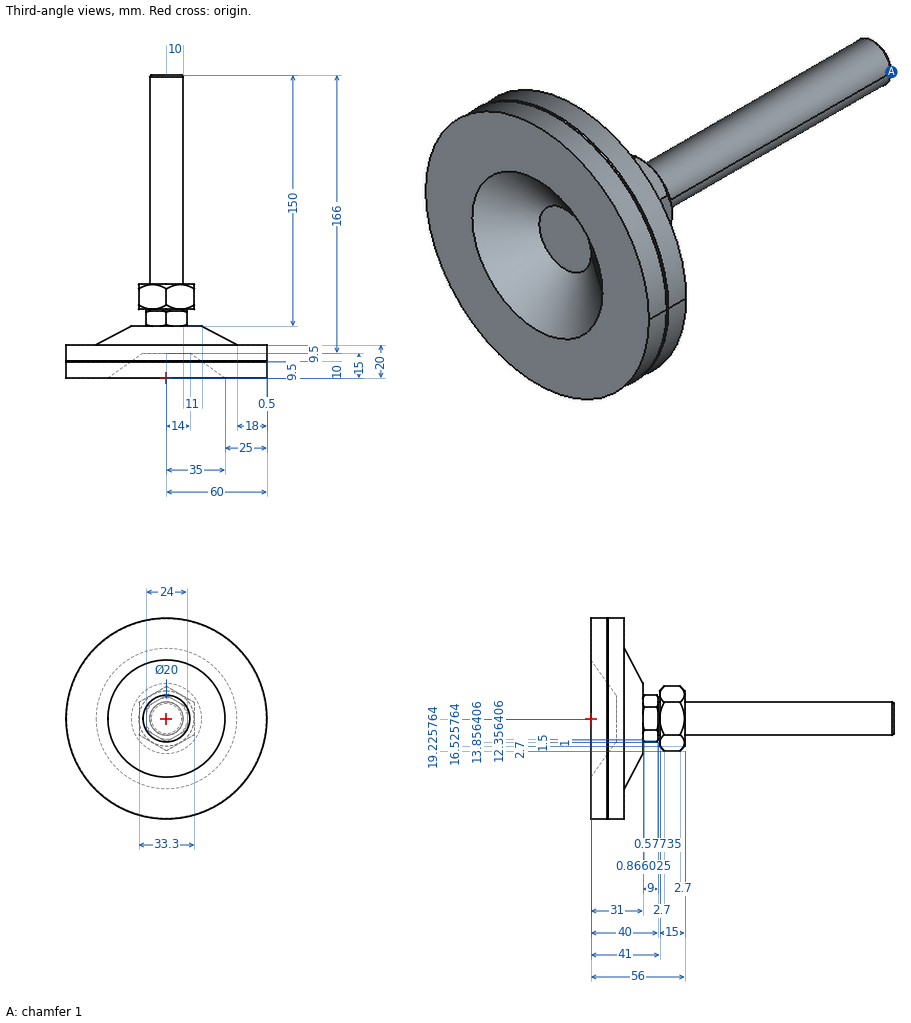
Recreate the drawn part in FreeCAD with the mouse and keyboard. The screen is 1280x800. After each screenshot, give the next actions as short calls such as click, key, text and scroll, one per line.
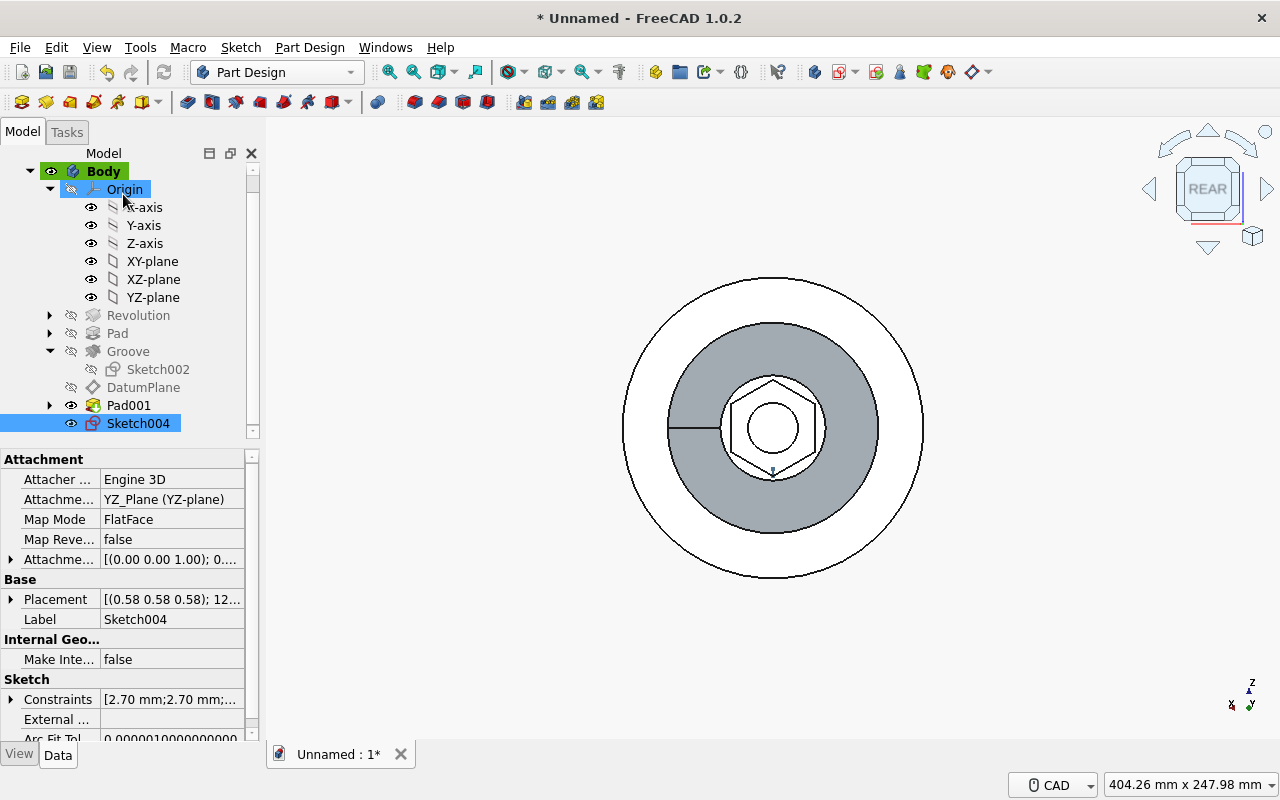
click(236, 102)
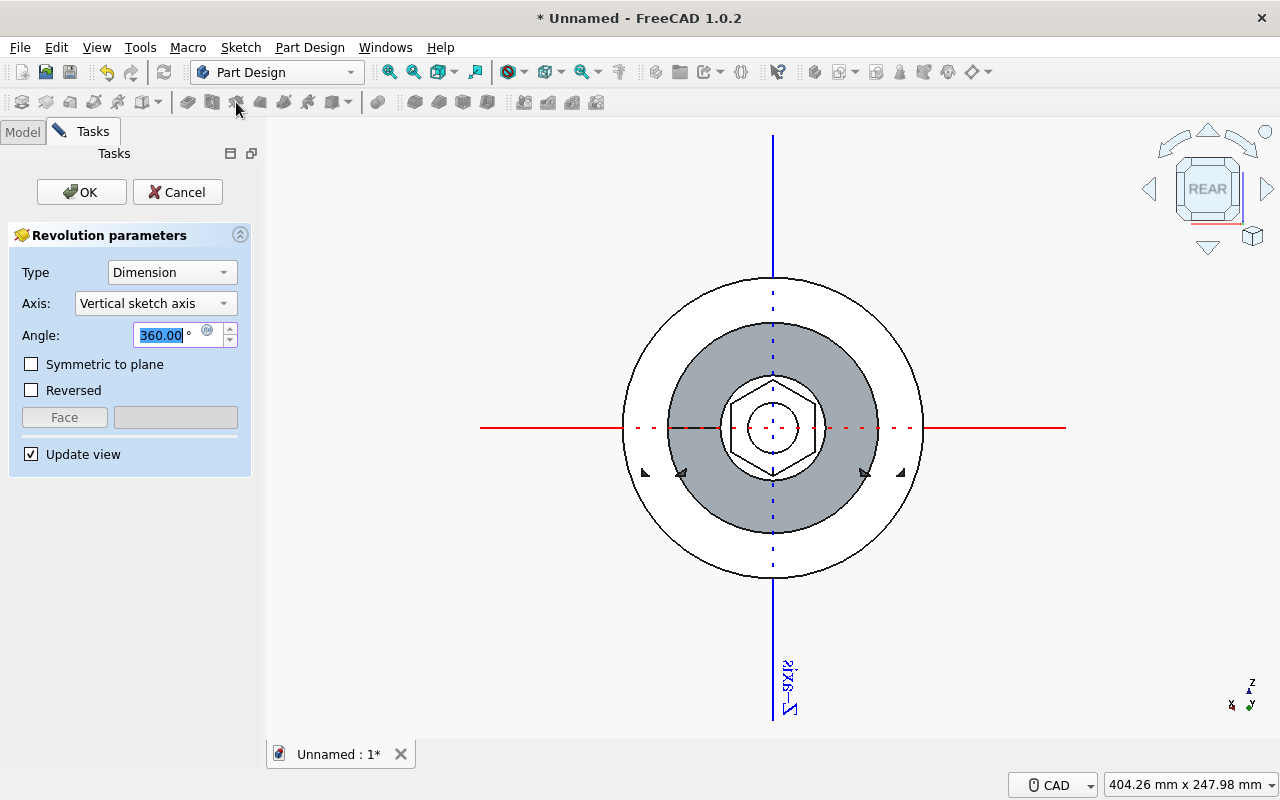
click(156, 304)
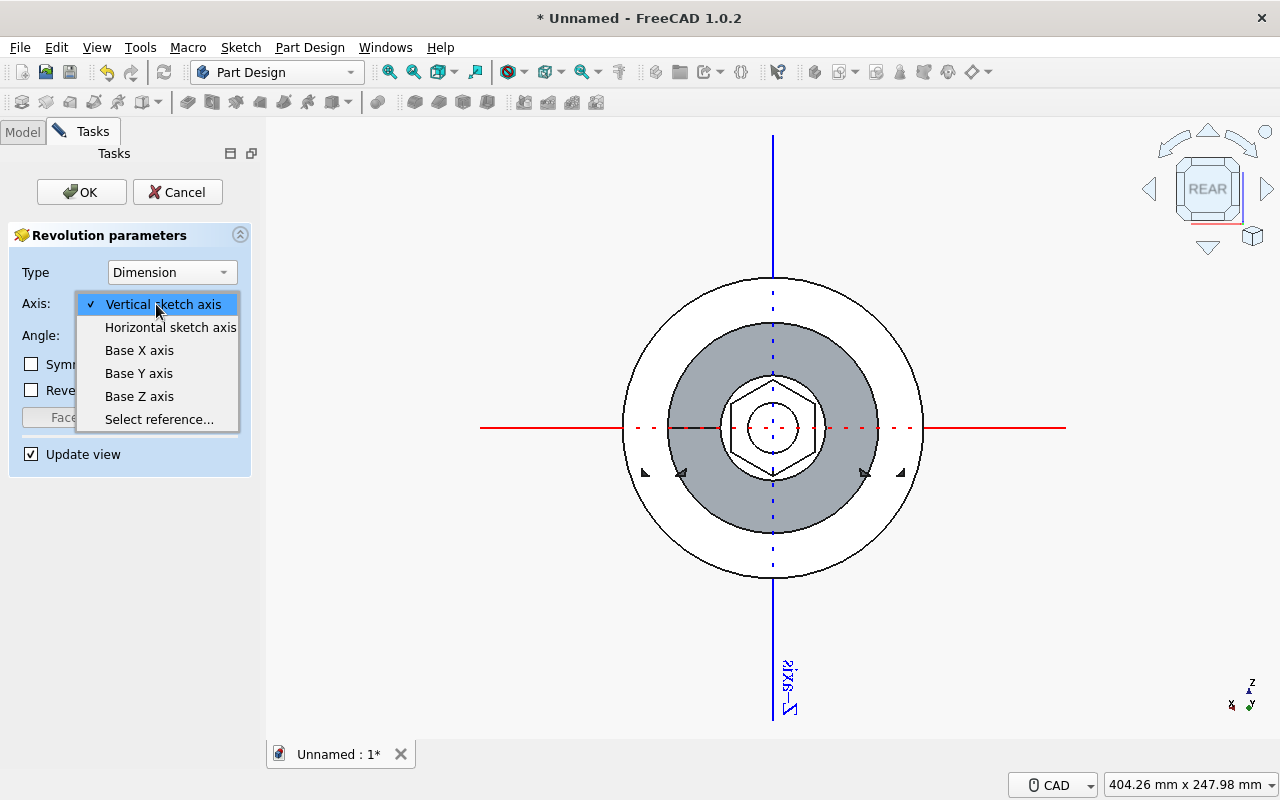
click(156, 328)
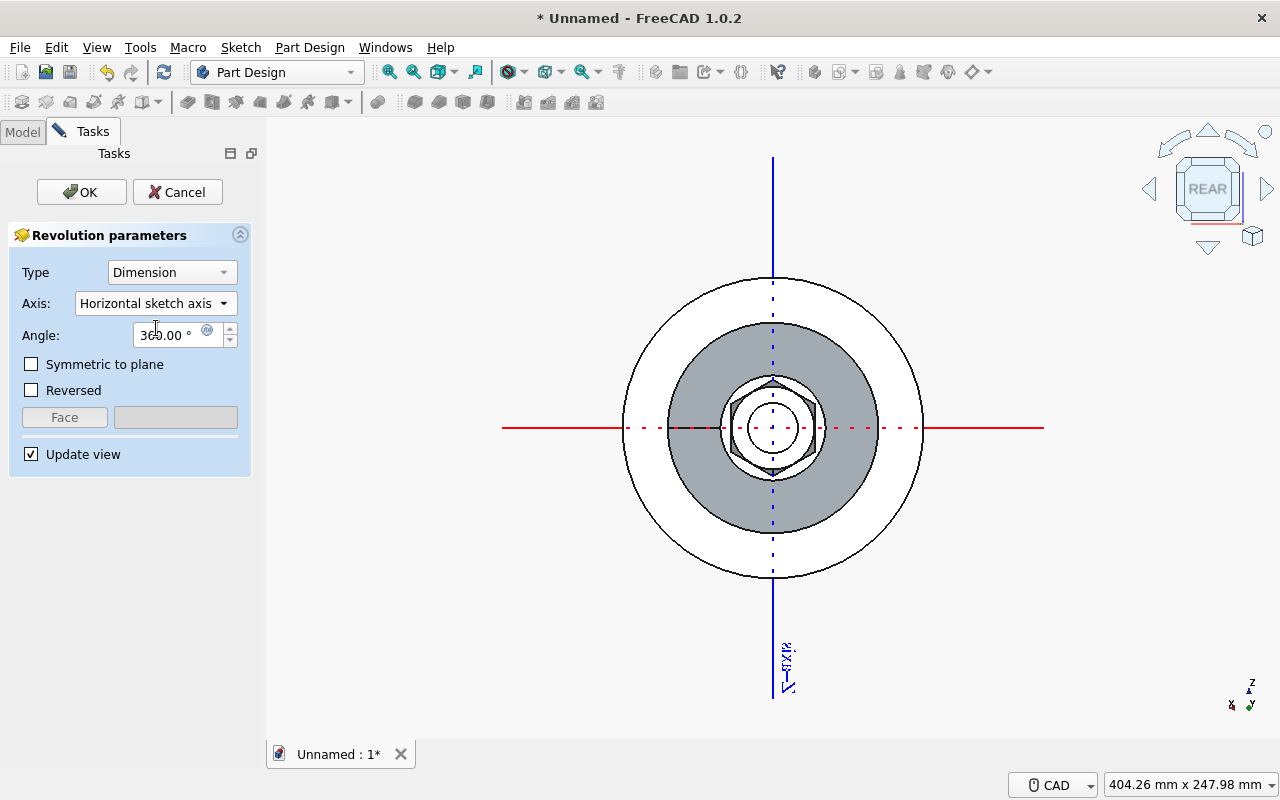
click(82, 192)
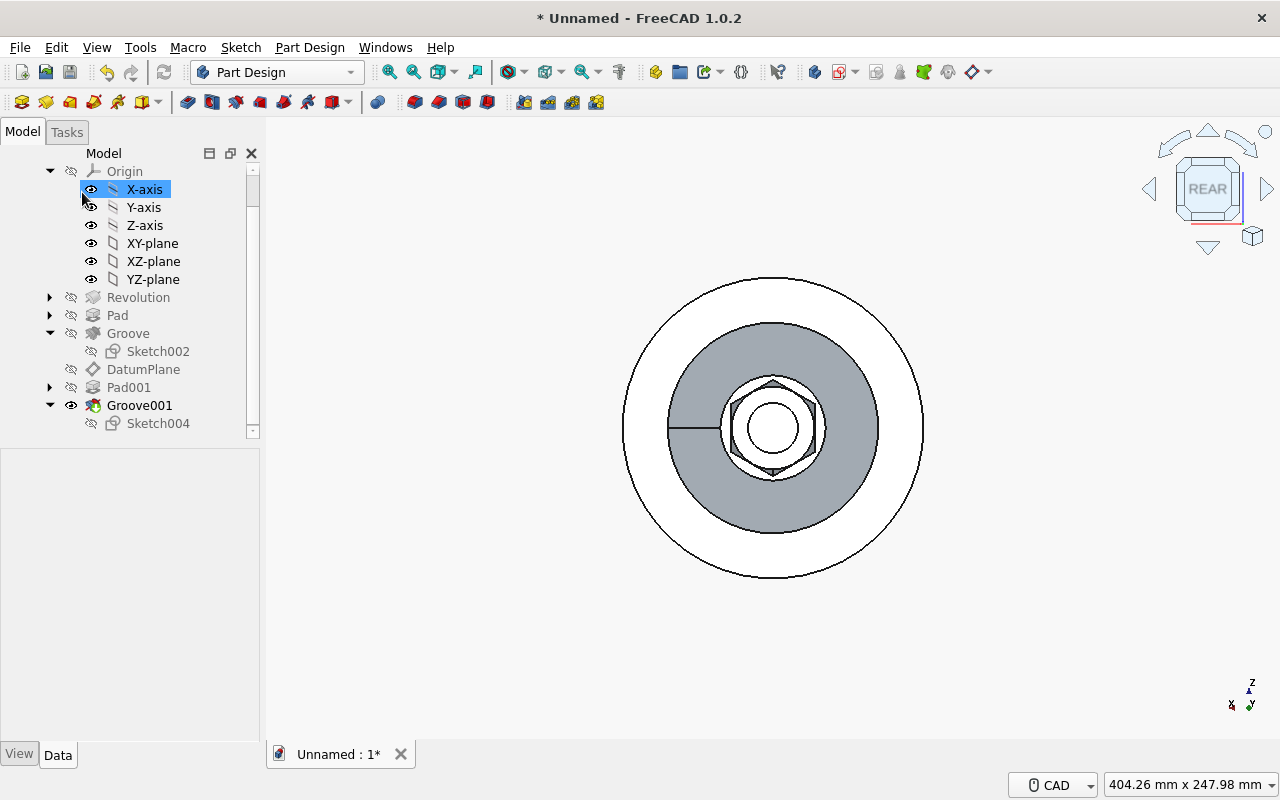
click(798, 427)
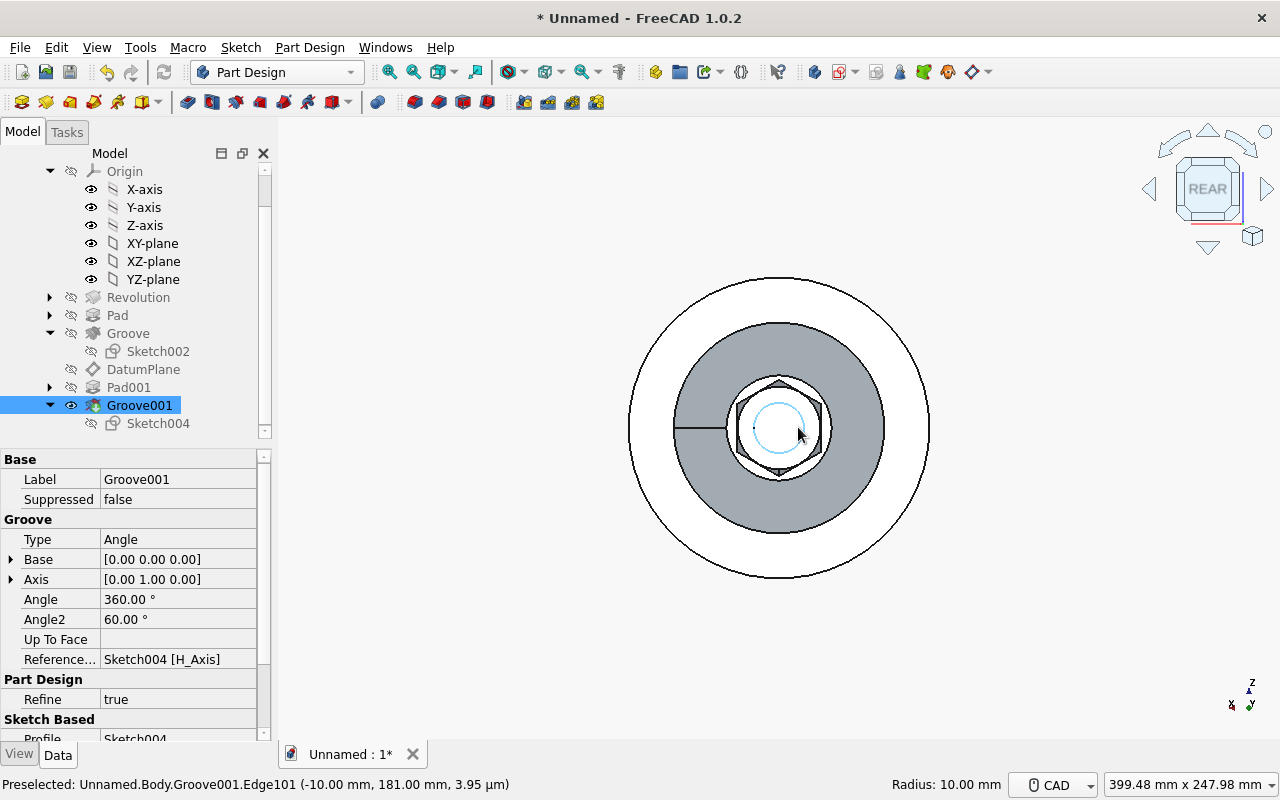
click(440, 102)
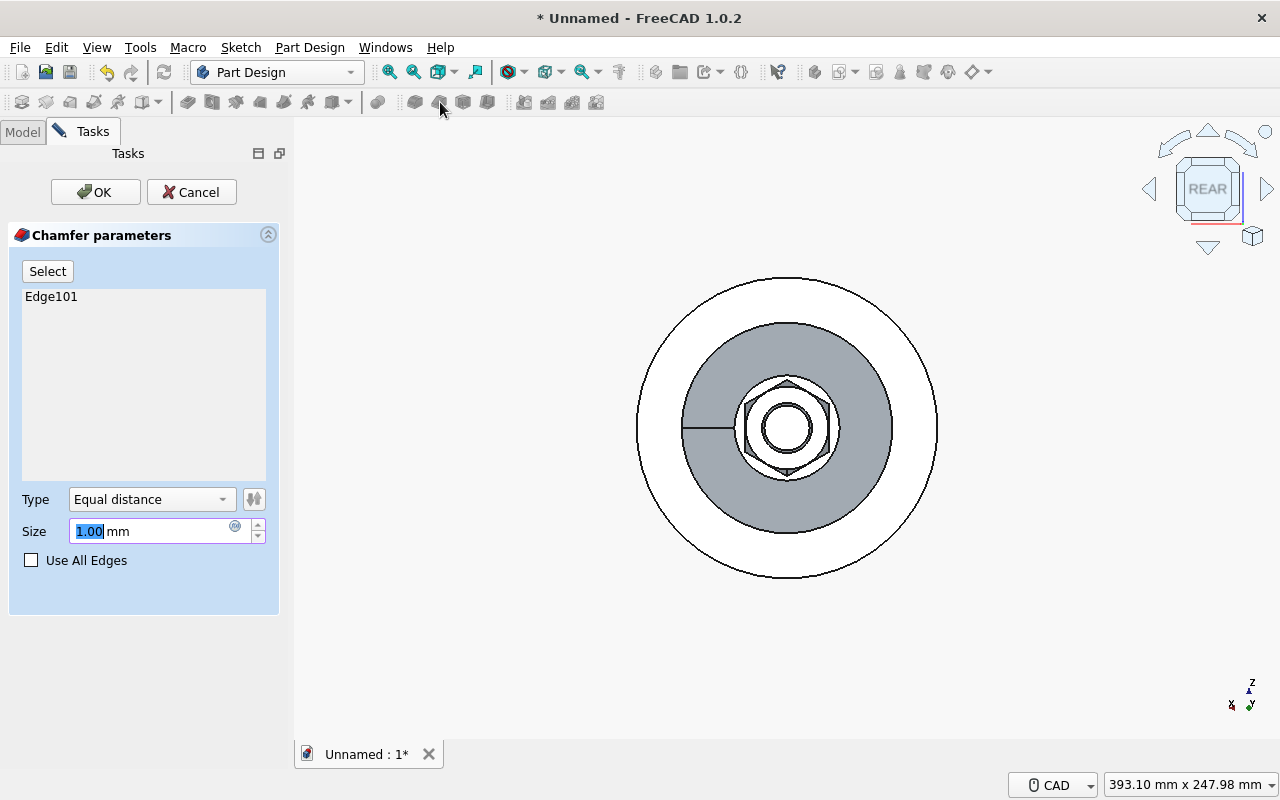
text(1)
key(Tab)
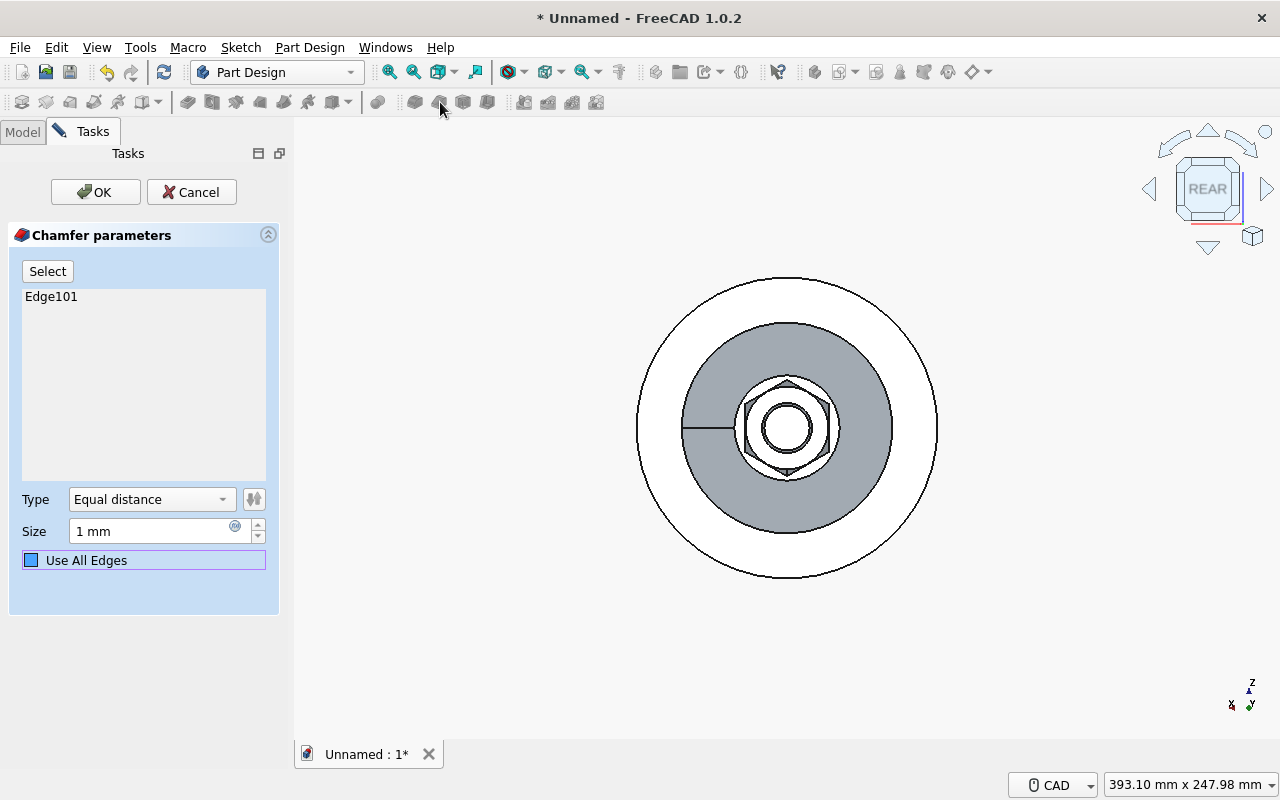
click(96, 192)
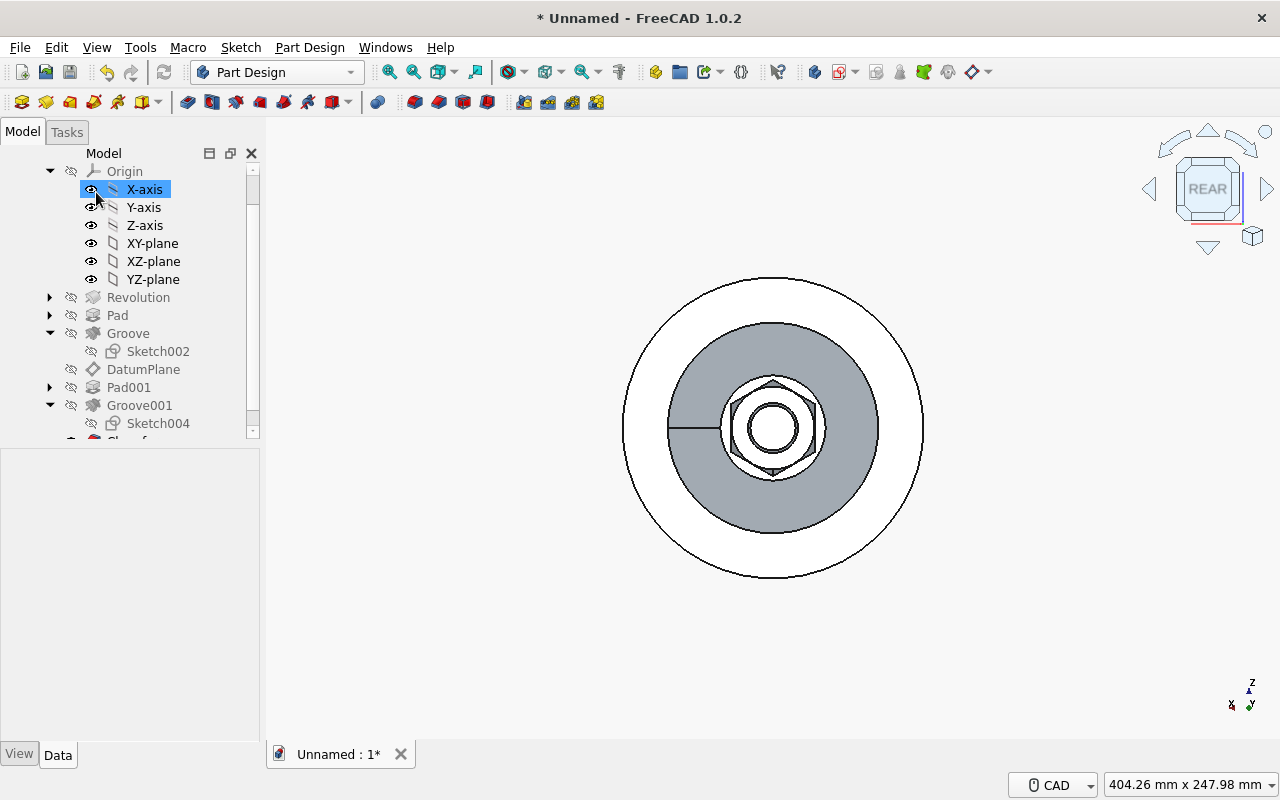
key(0)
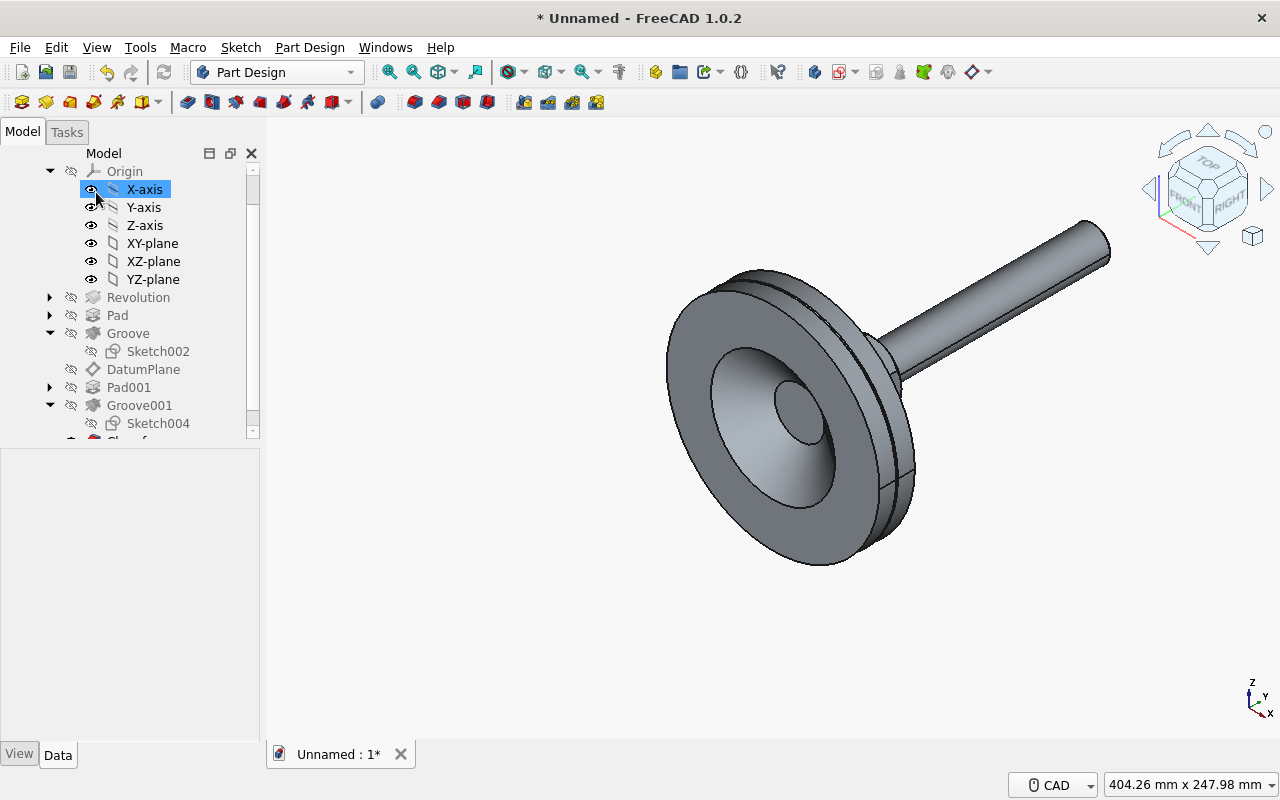
click(390, 72)